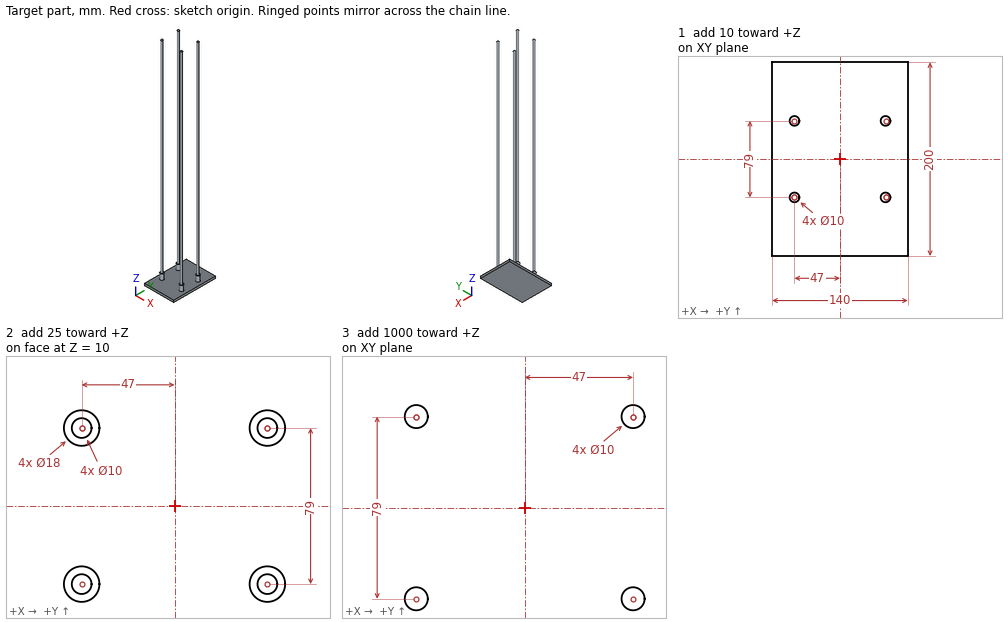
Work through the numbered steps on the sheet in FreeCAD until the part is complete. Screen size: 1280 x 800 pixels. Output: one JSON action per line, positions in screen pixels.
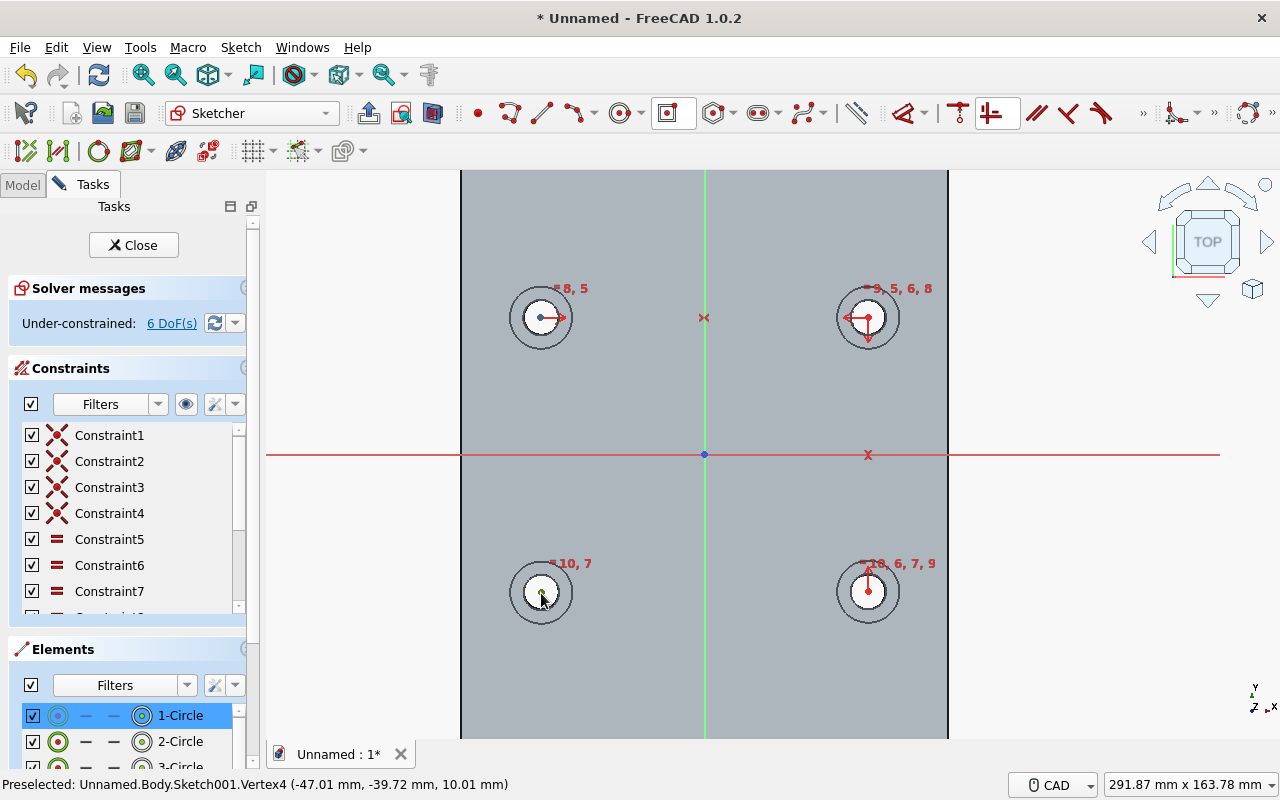
{"action": "left_click", "coordinate": [353, 455]}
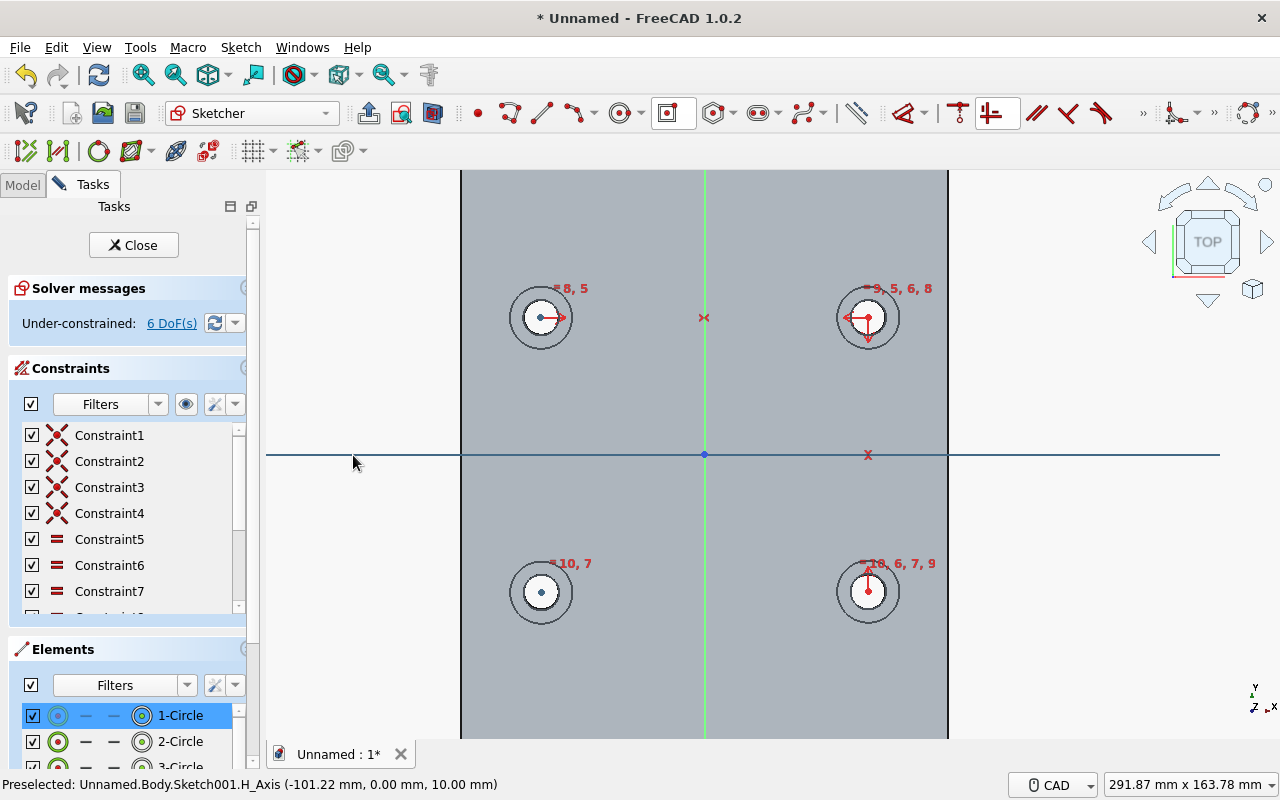
{"action": "key", "text": "s"}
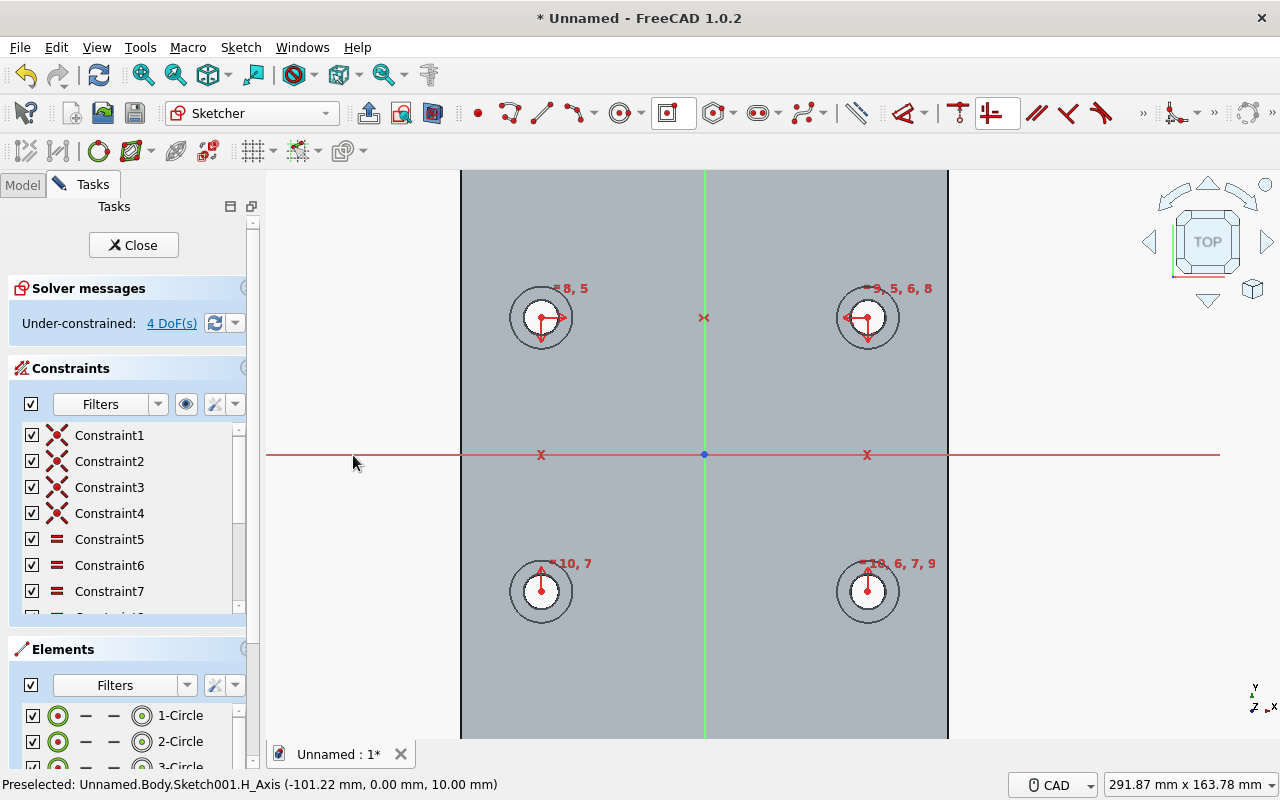
{"action": "left_click", "coordinate": [904, 114]}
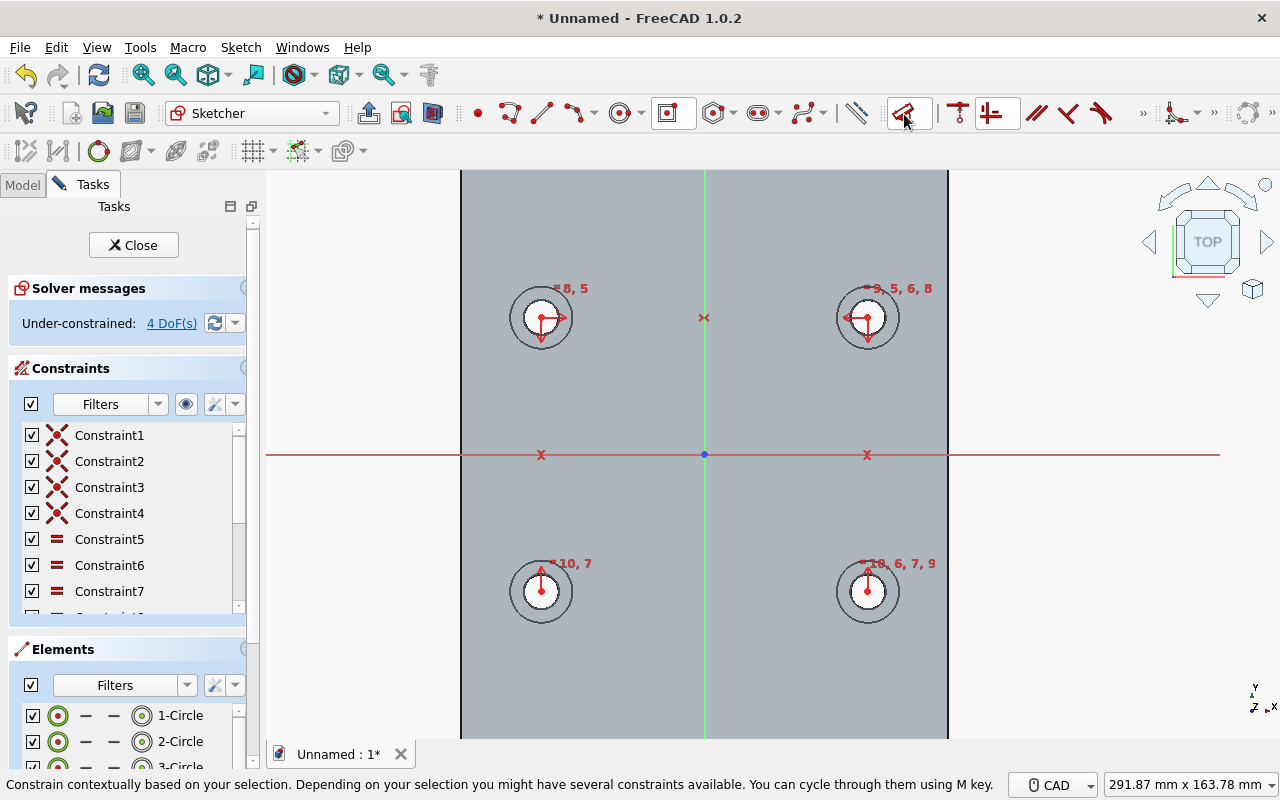
{"action": "left_click", "coordinate": [563, 296]}
{"action": "left_click", "coordinate": [586, 273]}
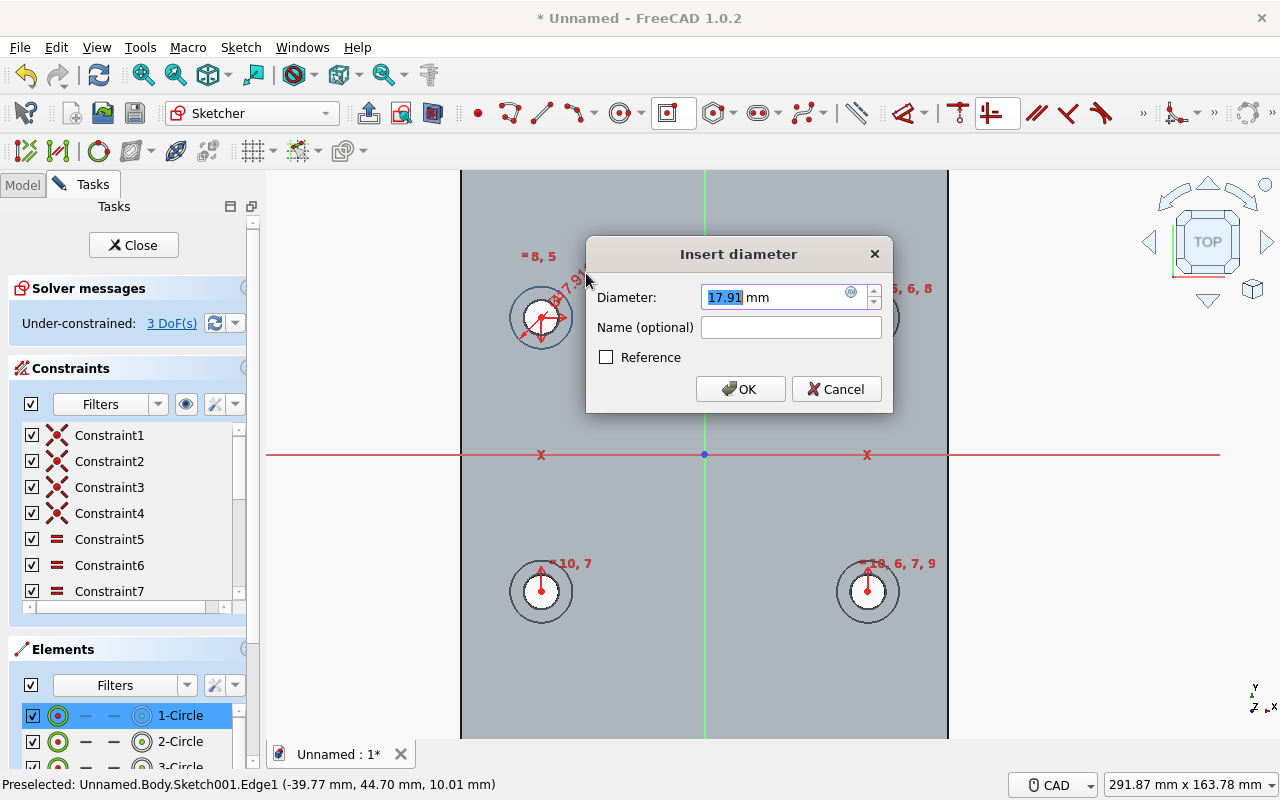
{"action": "type", "text": "18"}
{"action": "key", "text": "Return"}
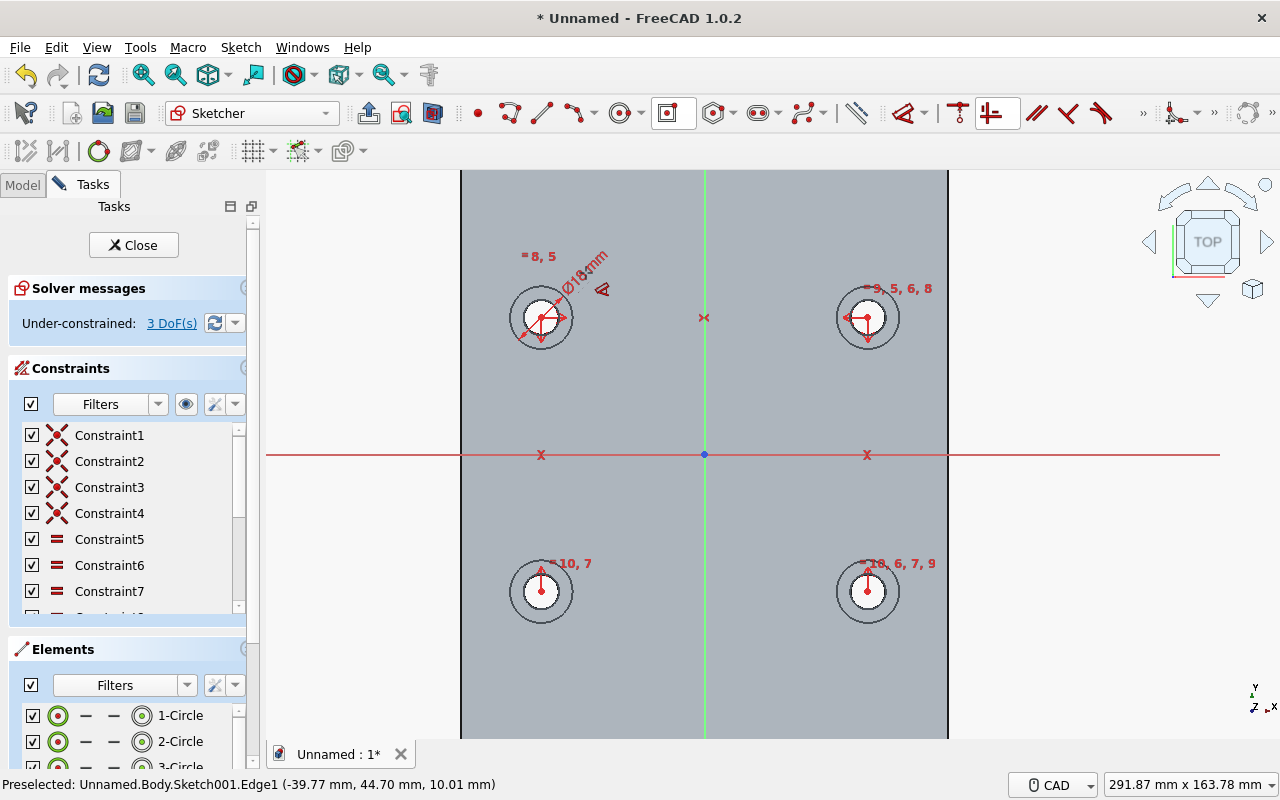
{"action": "left_click", "coordinate": [554, 305]}
{"action": "left_click", "coordinate": [589, 304]}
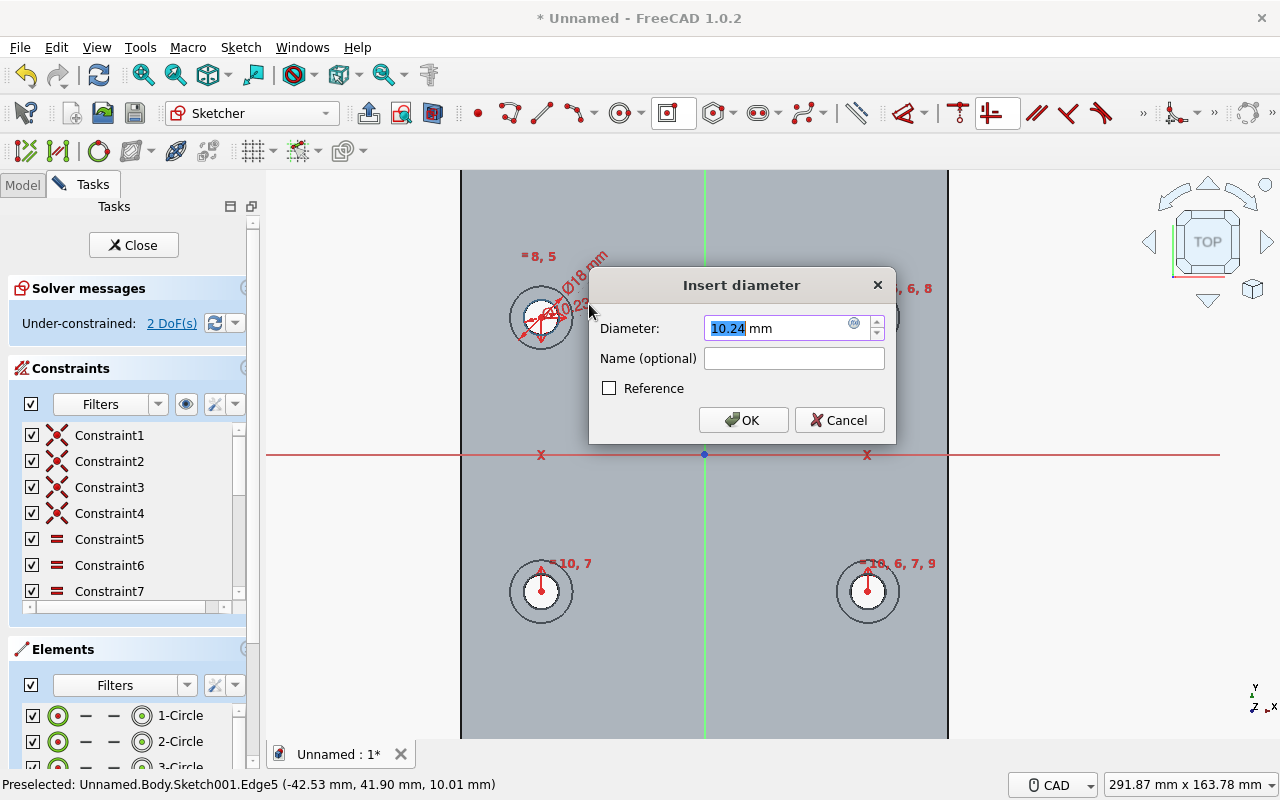
{"action": "type", "text": "10"}
{"action": "key", "text": "Return"}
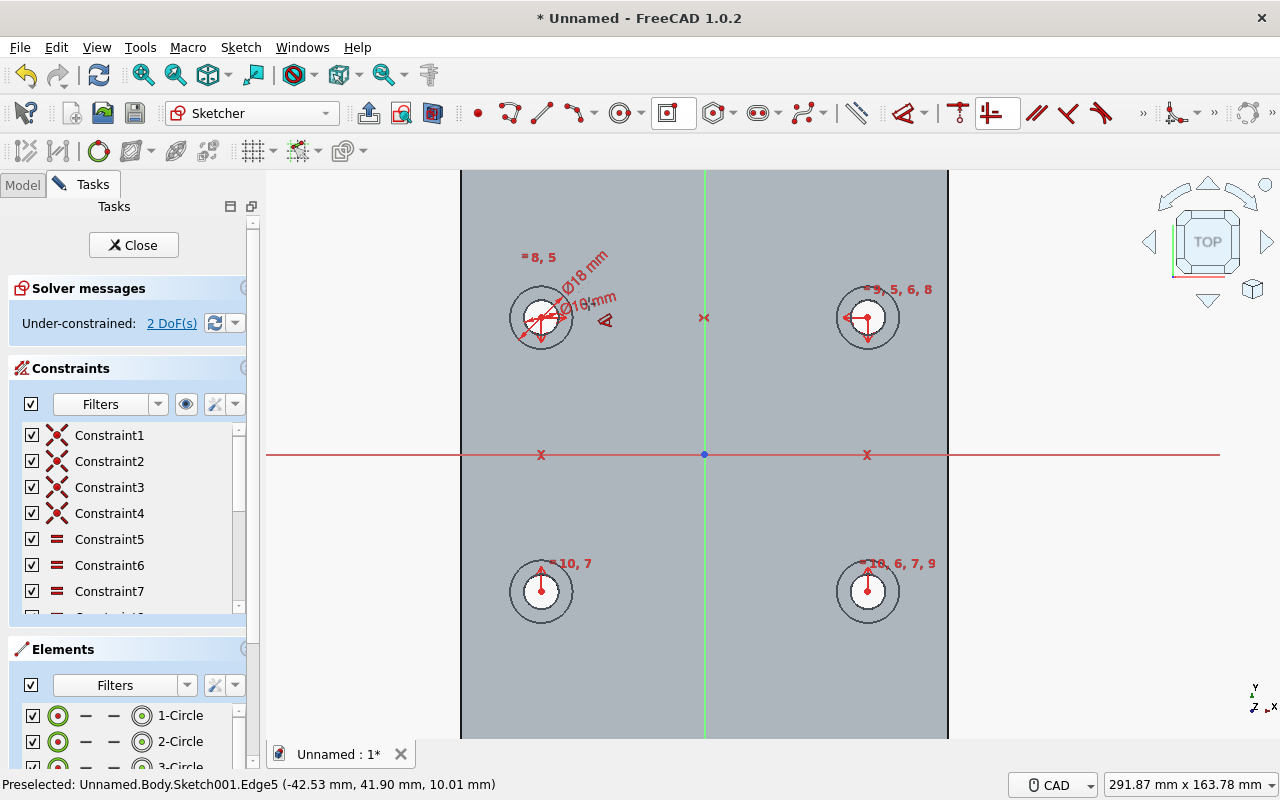
{"action": "left_click", "coordinate": [541, 318]}
{"action": "left_click", "coordinate": [661, 284]}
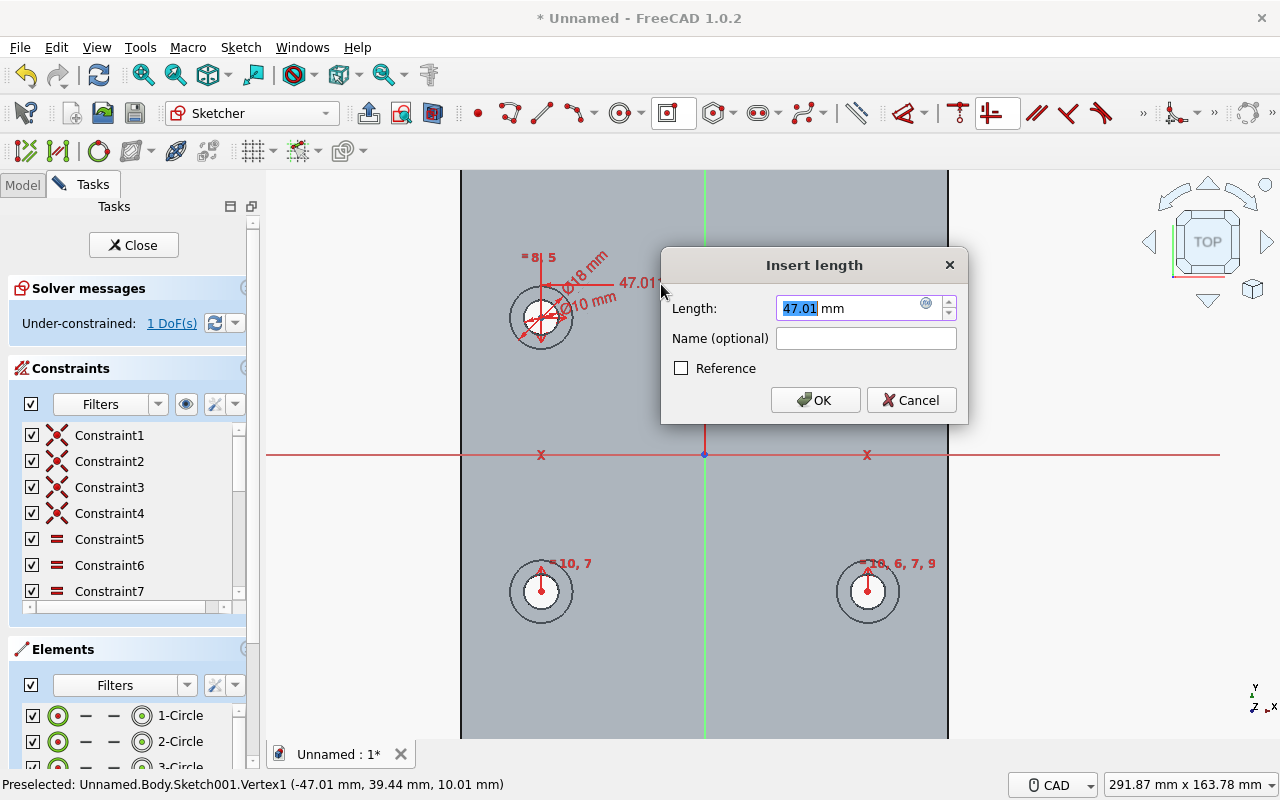
{"action": "type", "text": "47"}
{"action": "key", "text": "Return"}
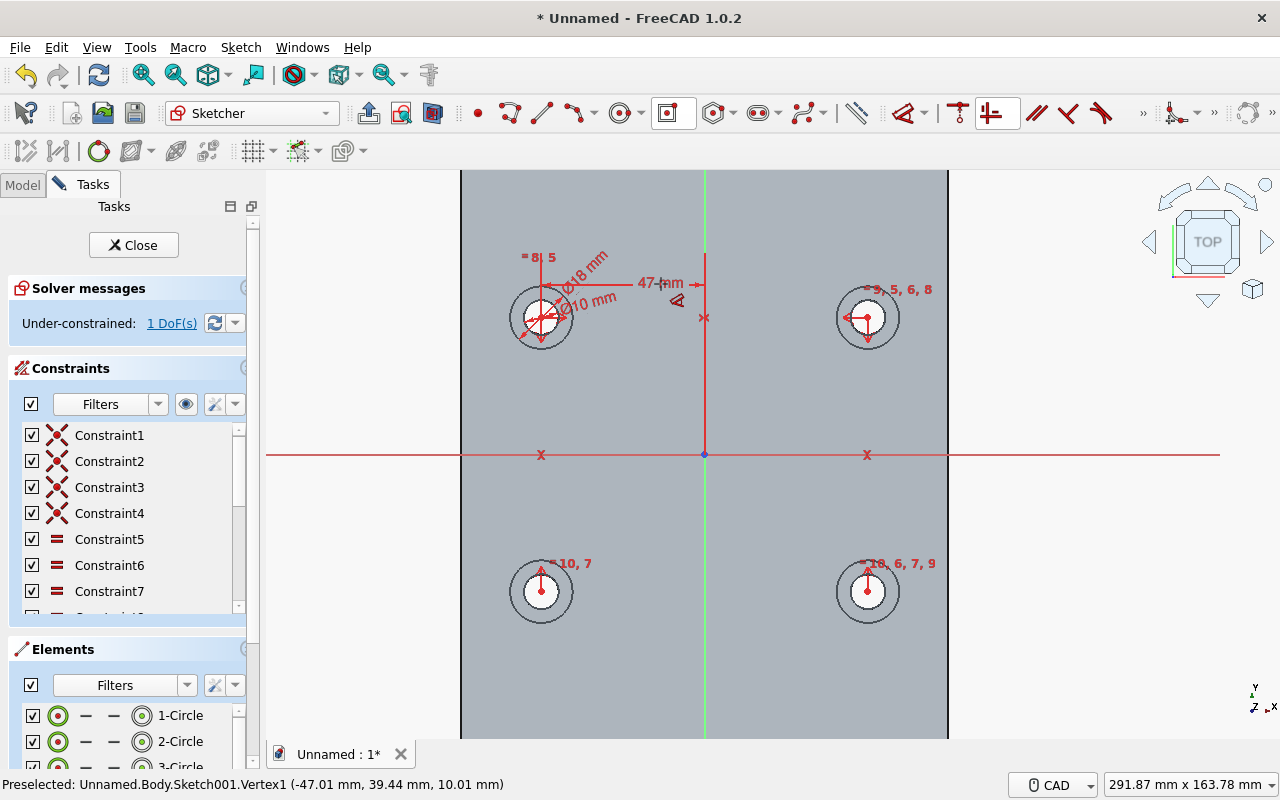
{"action": "left_click", "coordinate": [868, 318]}